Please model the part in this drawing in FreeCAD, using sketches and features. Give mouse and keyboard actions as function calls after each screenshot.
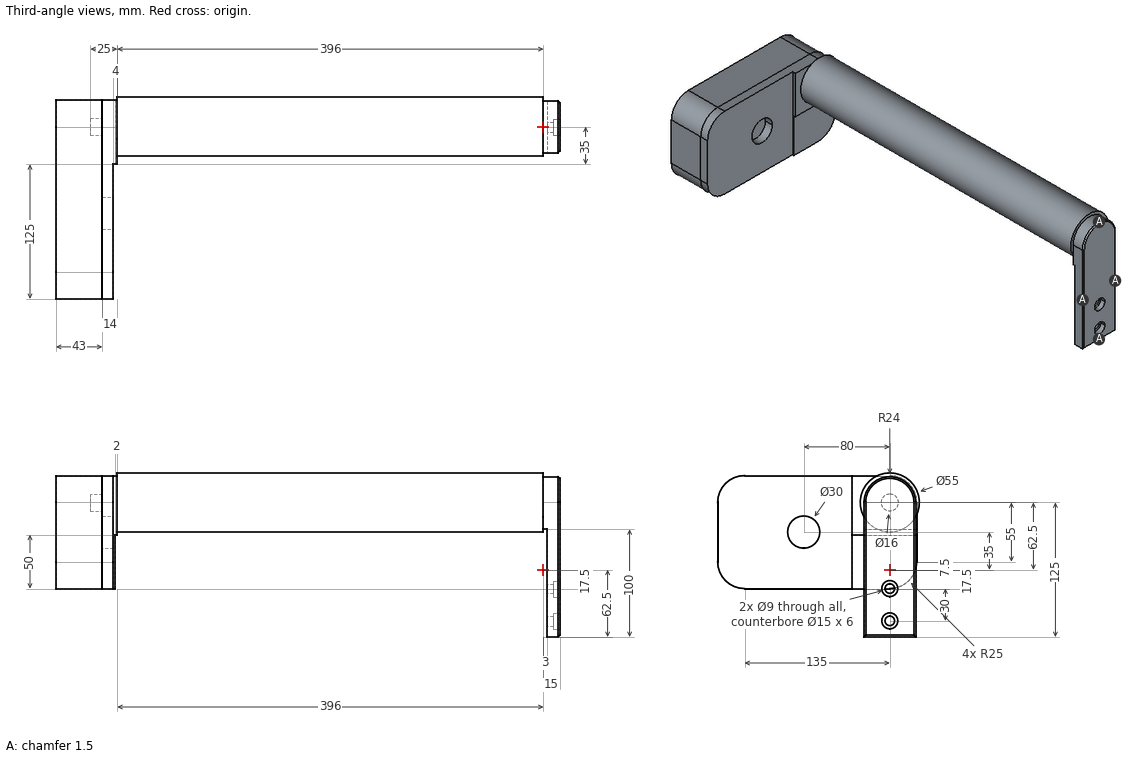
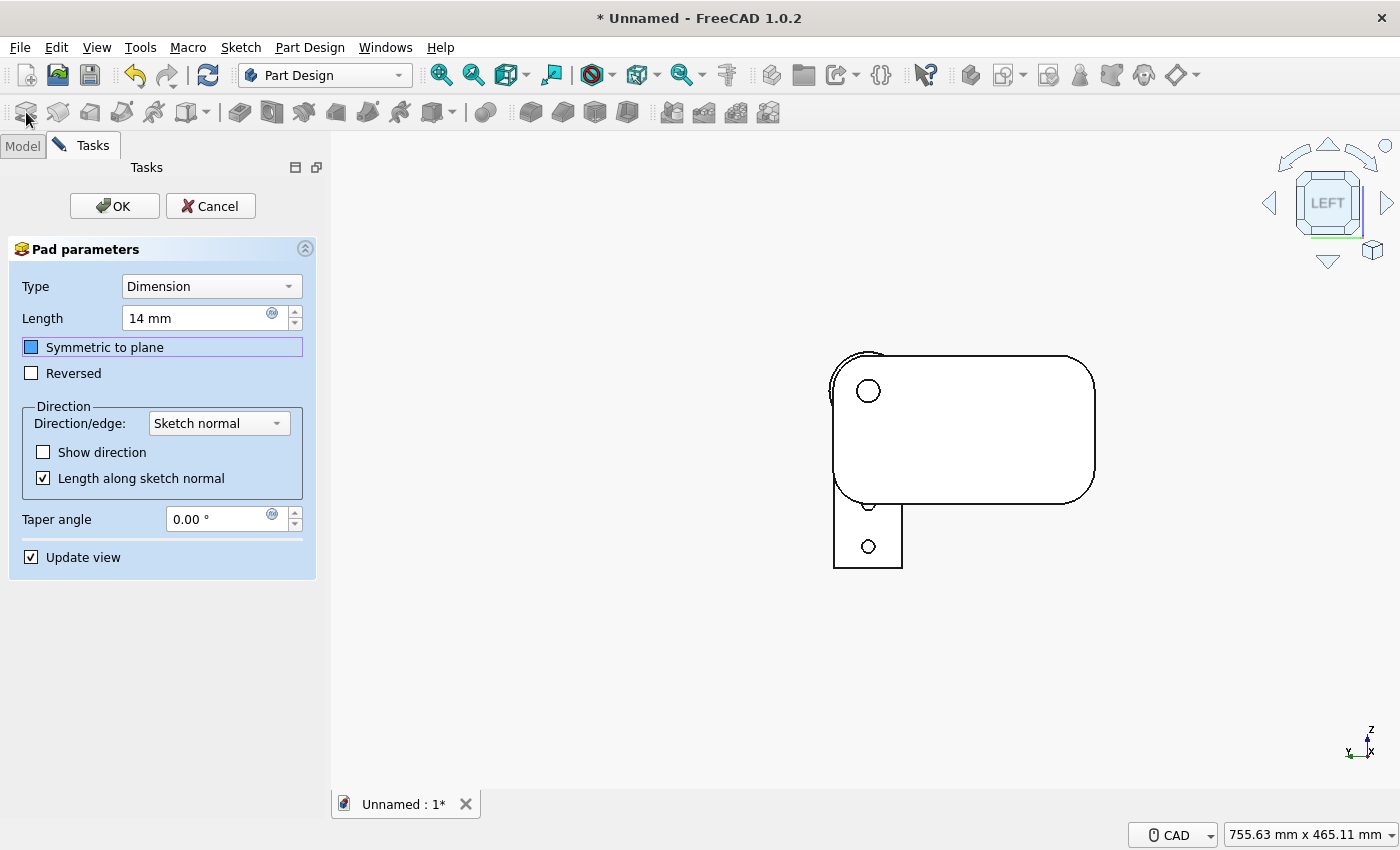
click(115, 206)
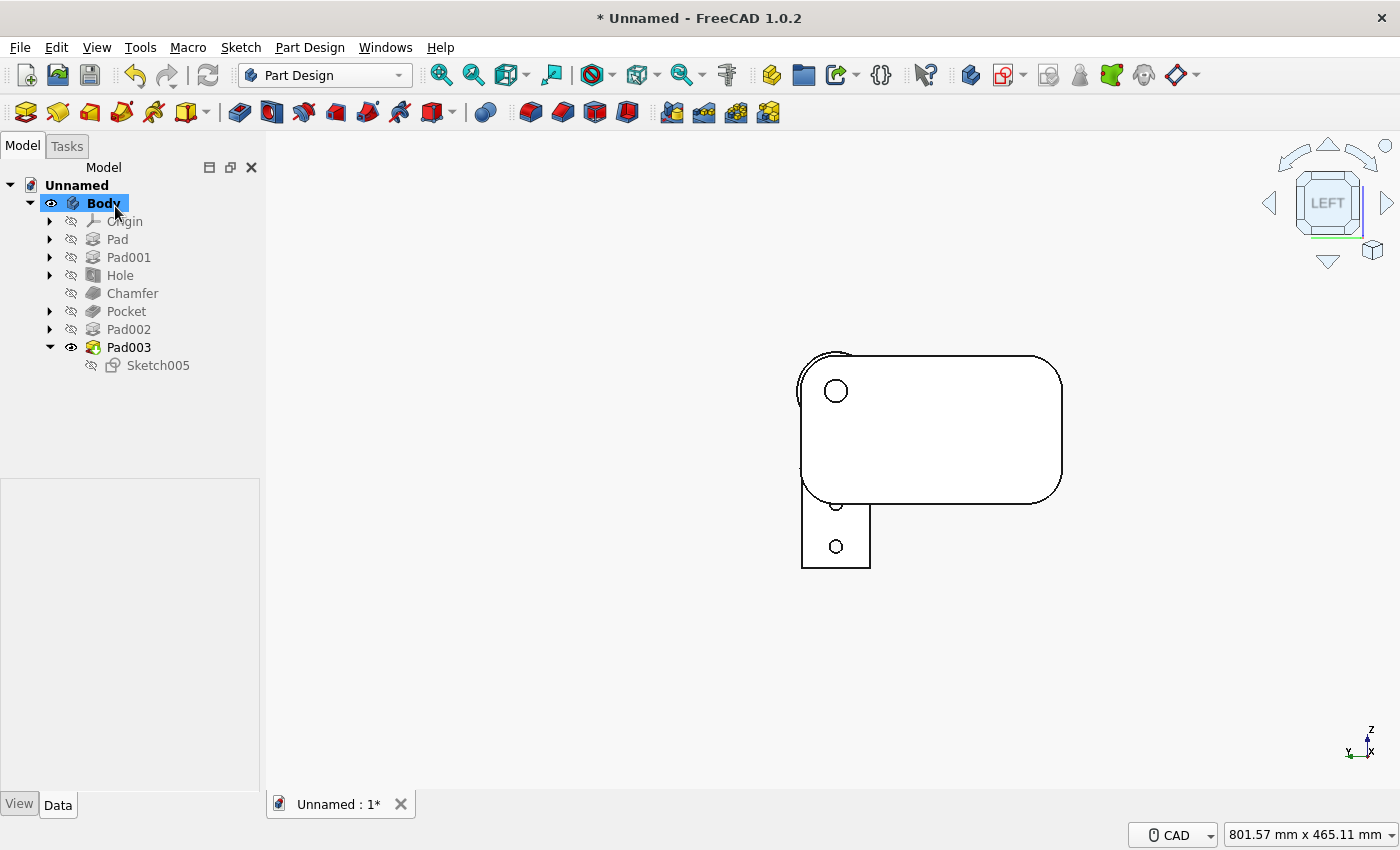
key(v)
key(f)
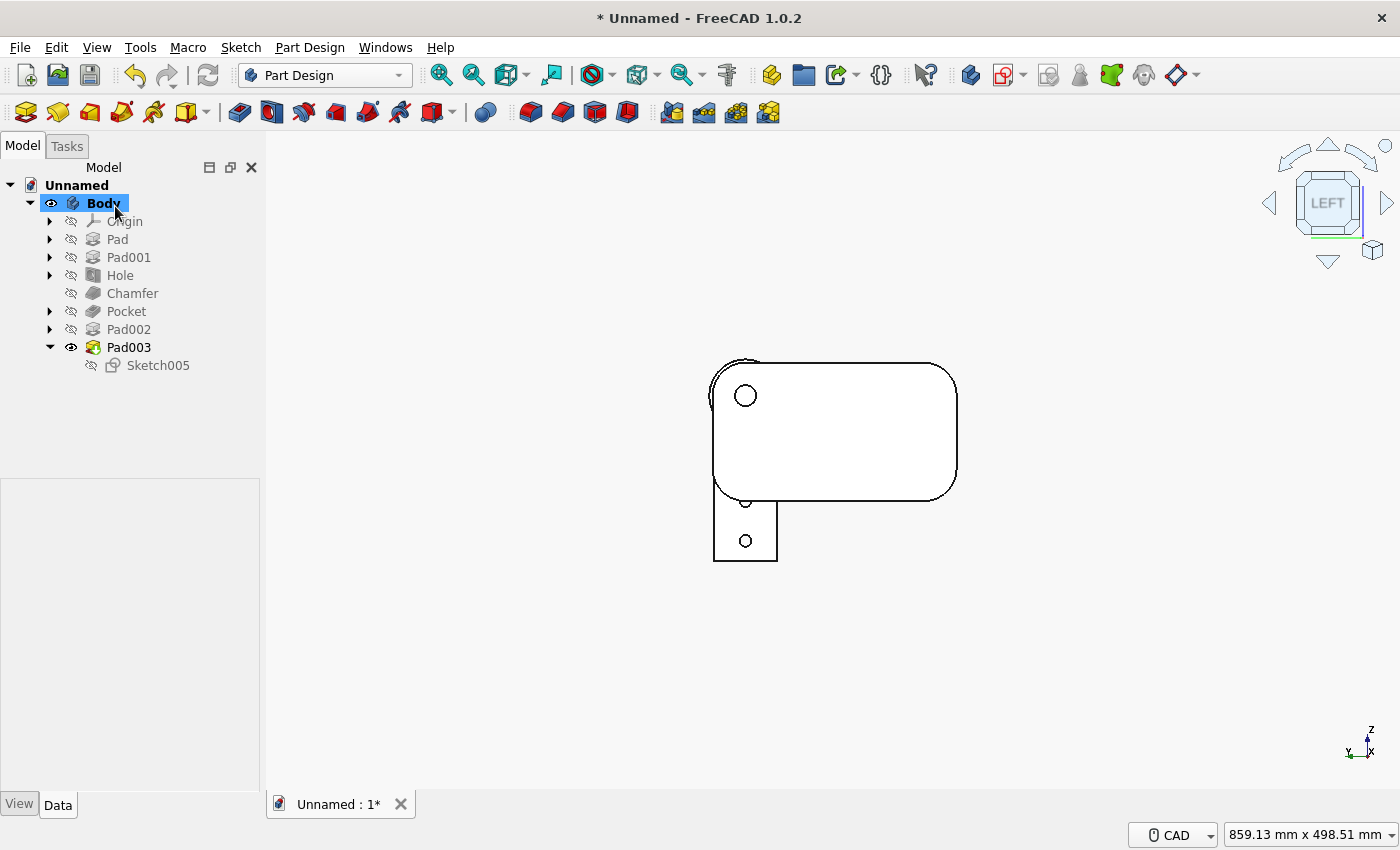
key(5)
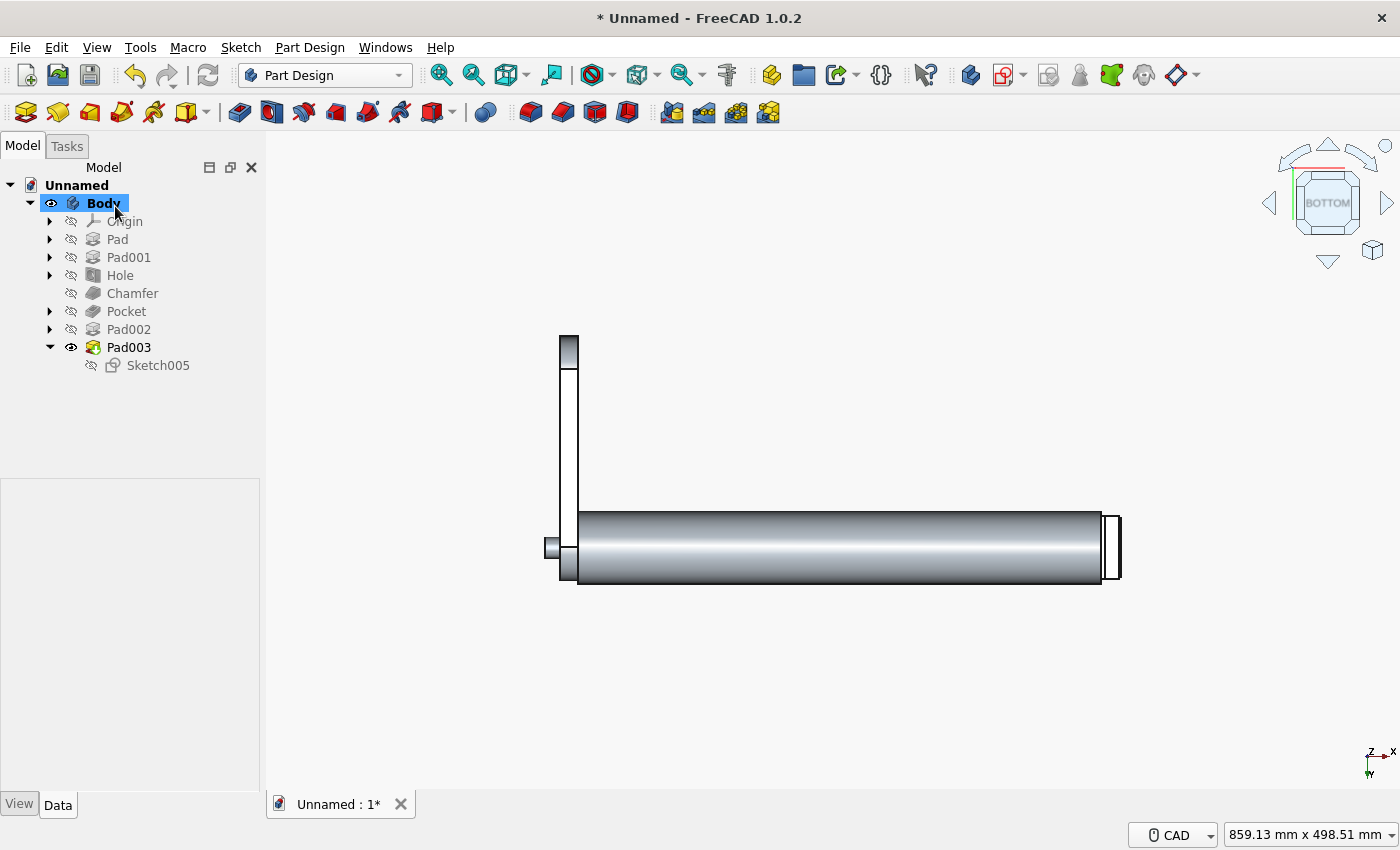
click(569, 534)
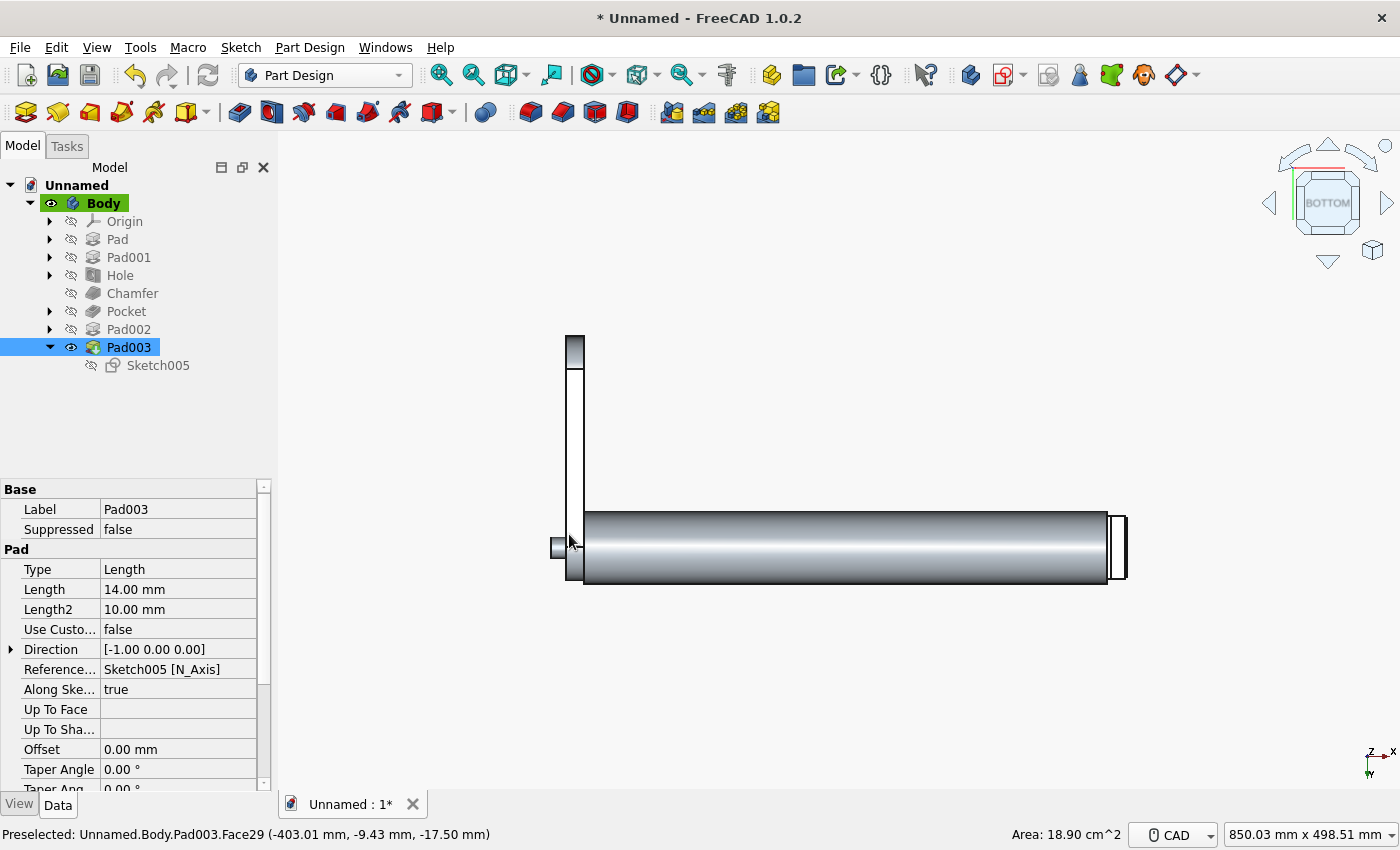
click(1004, 76)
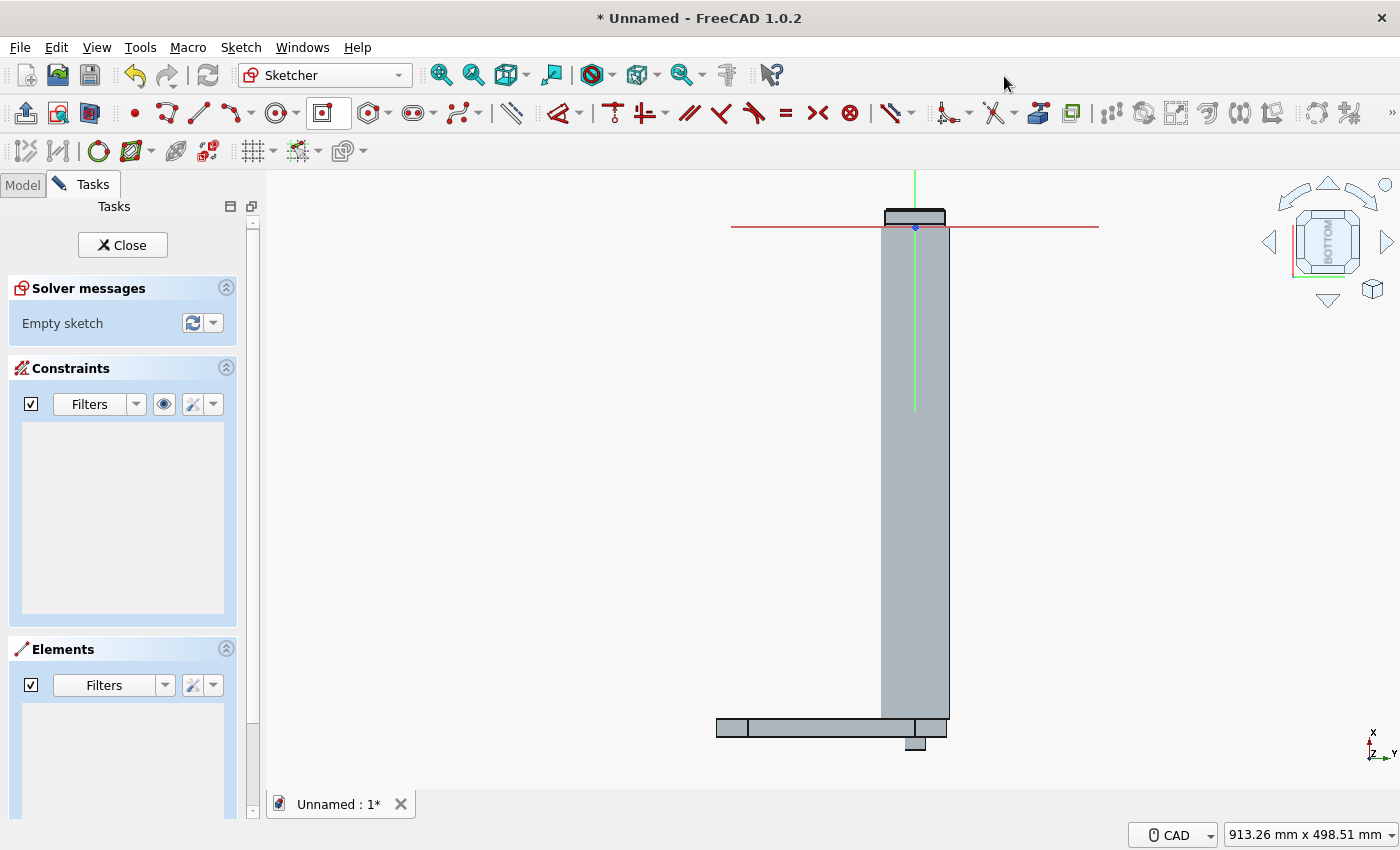
key(q)
key(s)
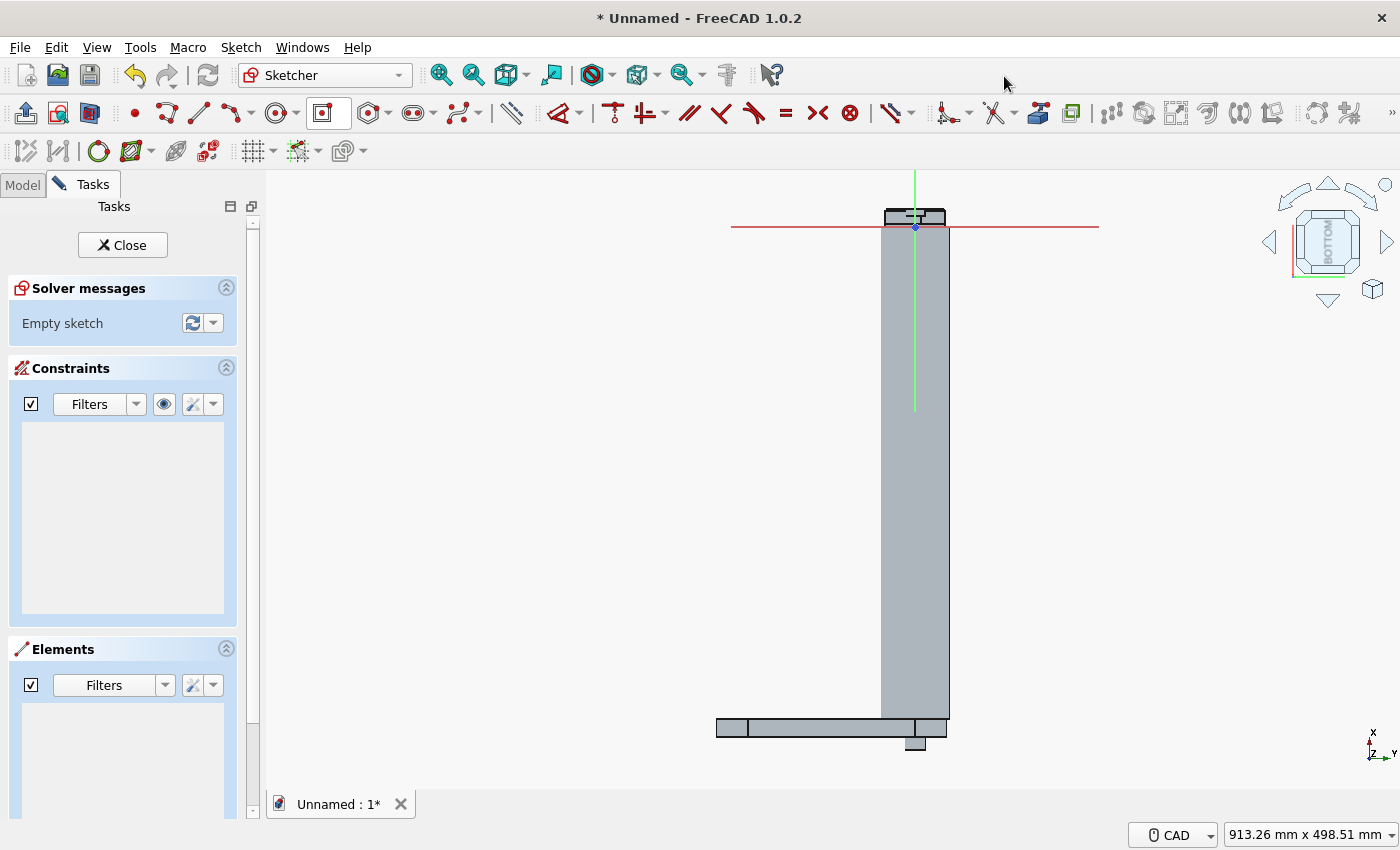
scroll(804, 761, up, 7)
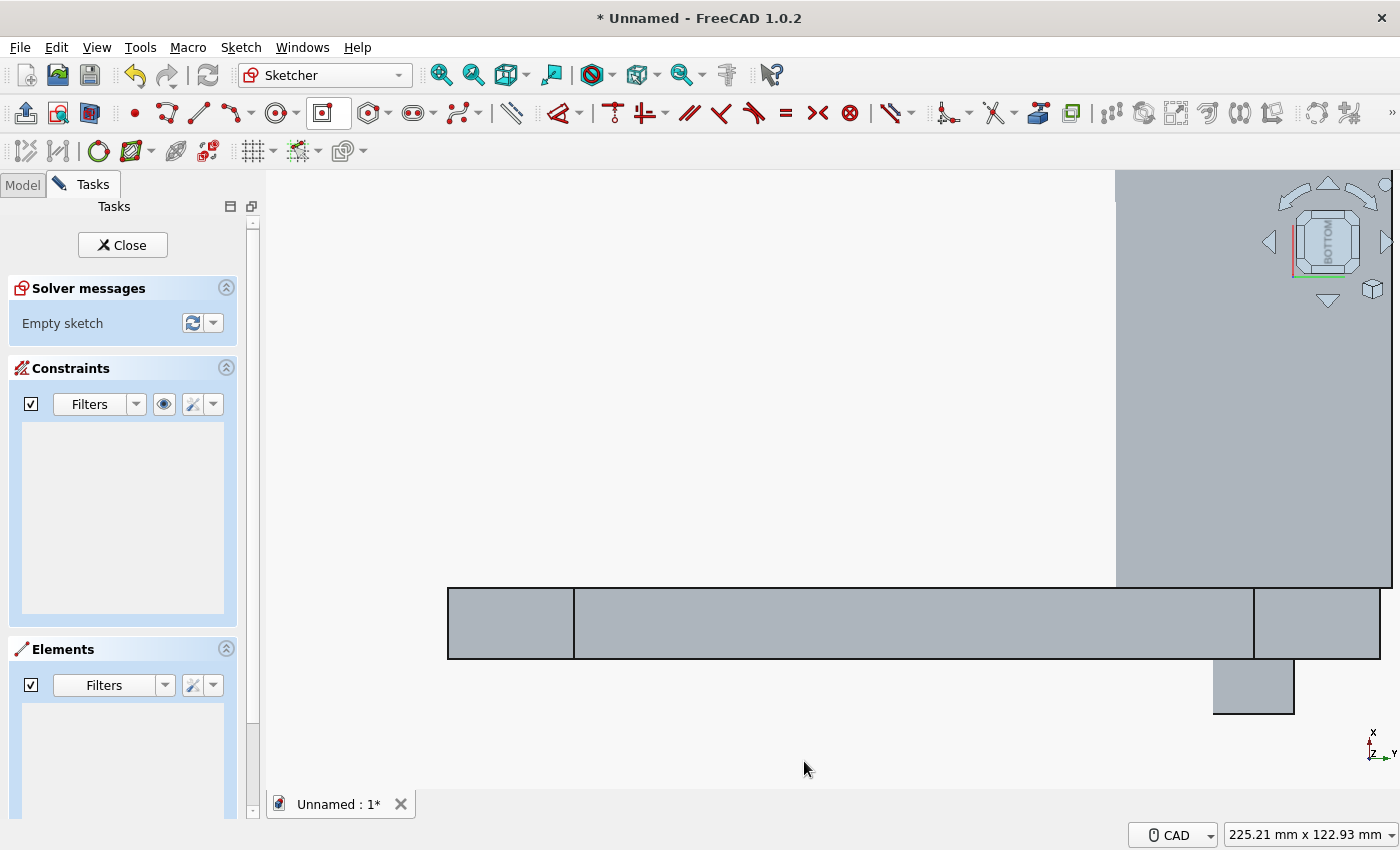
key(g)
key(r)